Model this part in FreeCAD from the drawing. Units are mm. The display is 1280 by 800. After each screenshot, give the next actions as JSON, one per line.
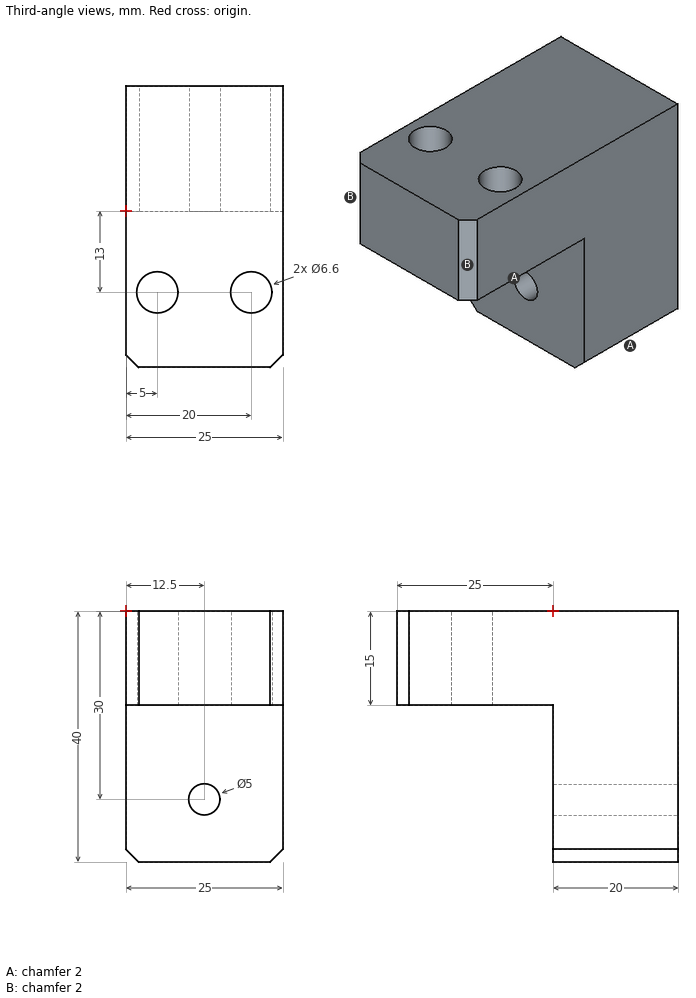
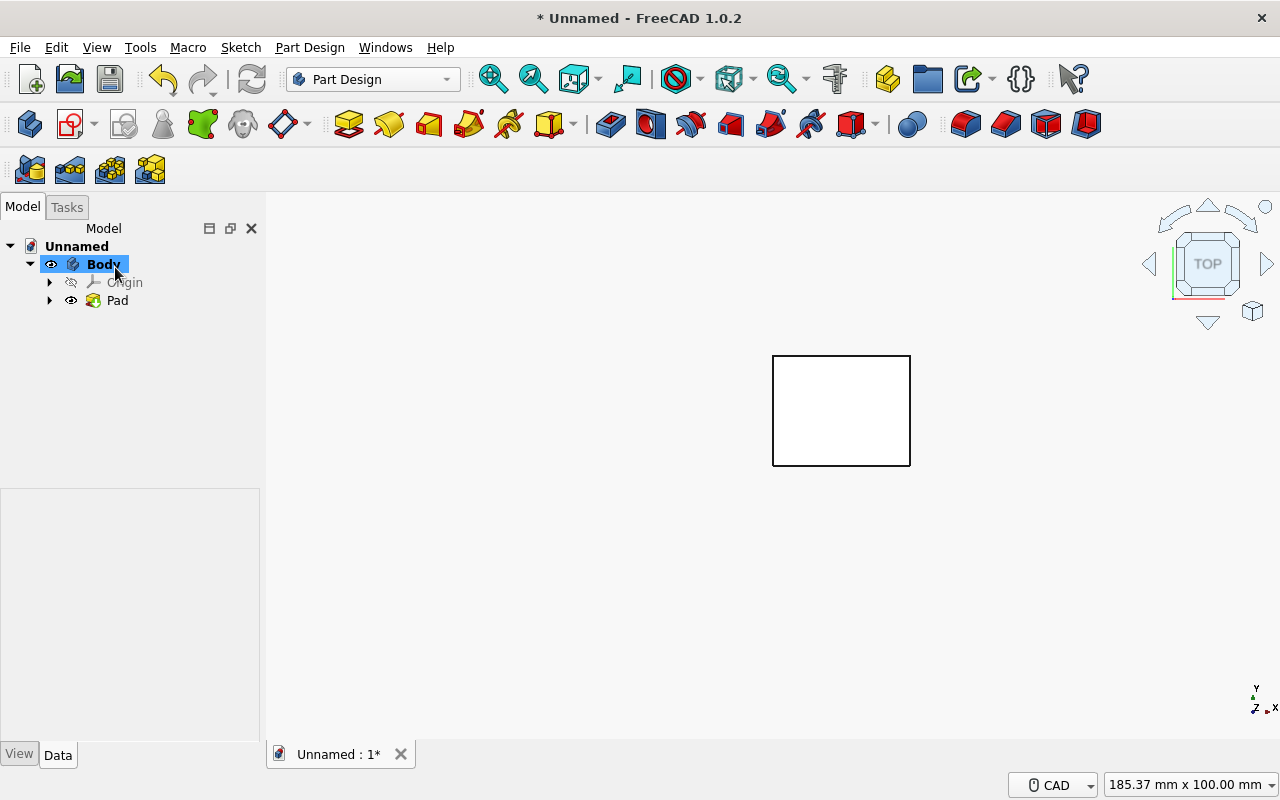
{"action": "key", "text": "v f"}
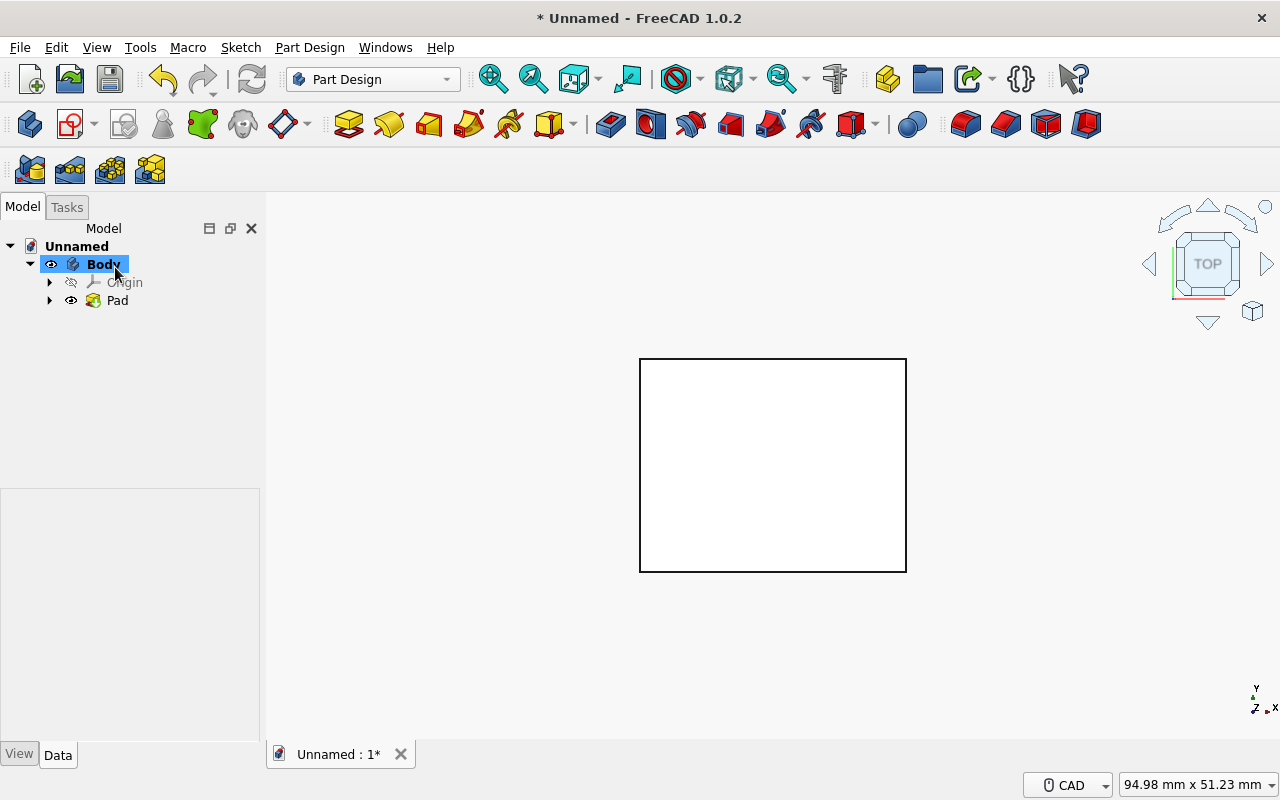
{"action": "key", "text": "1"}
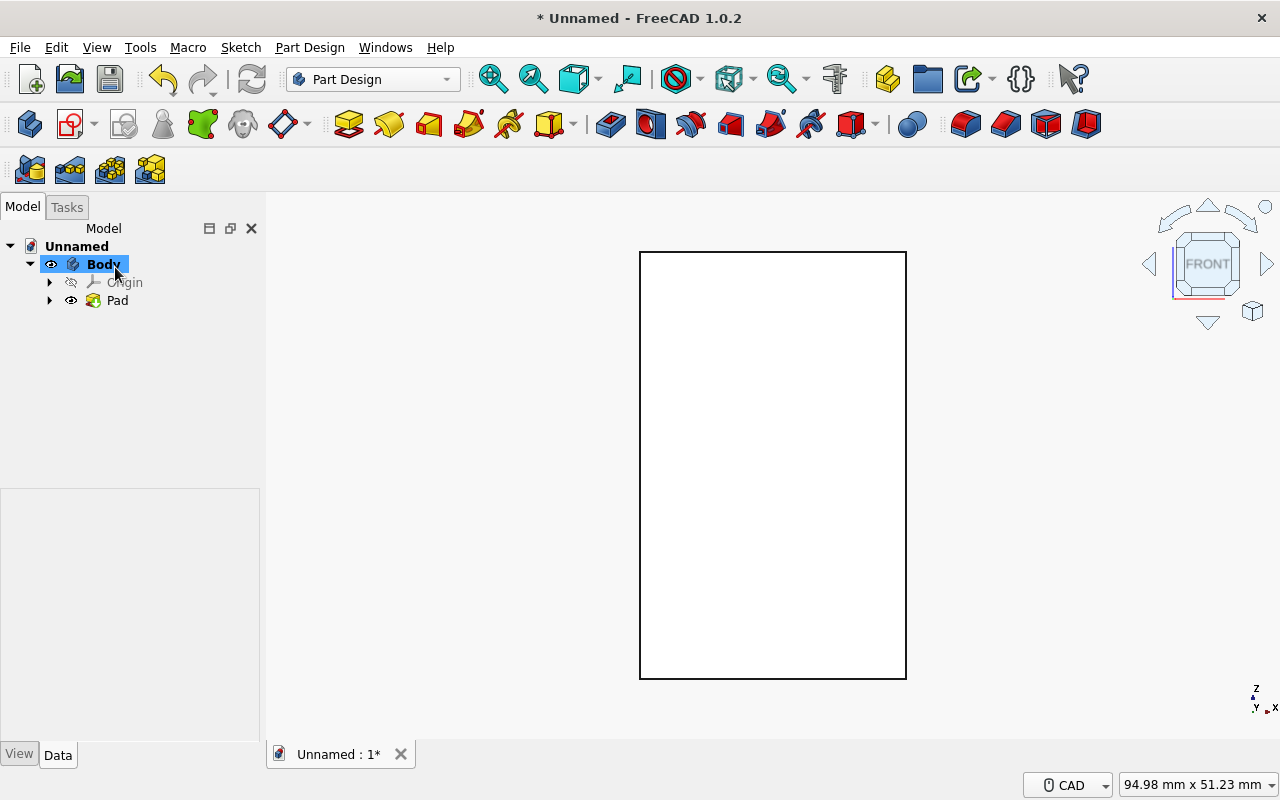
{"action": "key", "text": "3"}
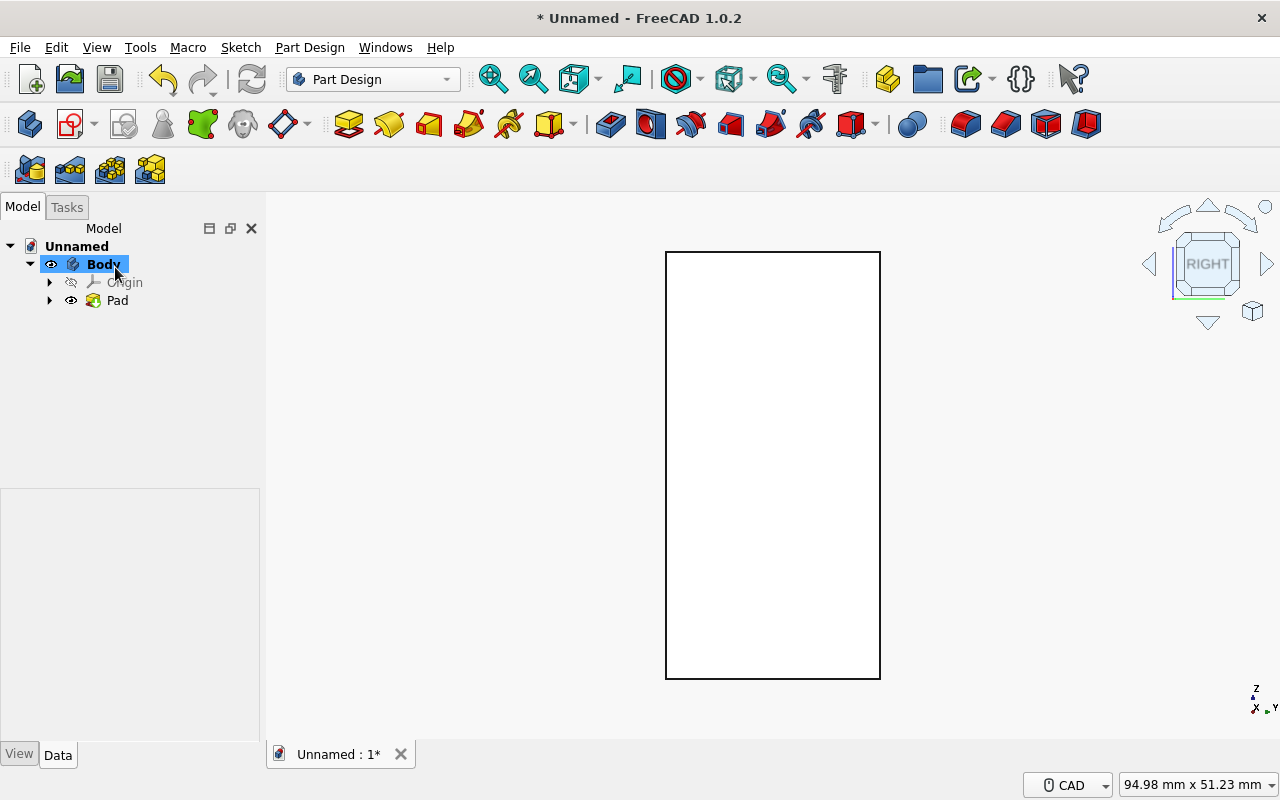
{"action": "left_click", "coordinate": [773, 678]}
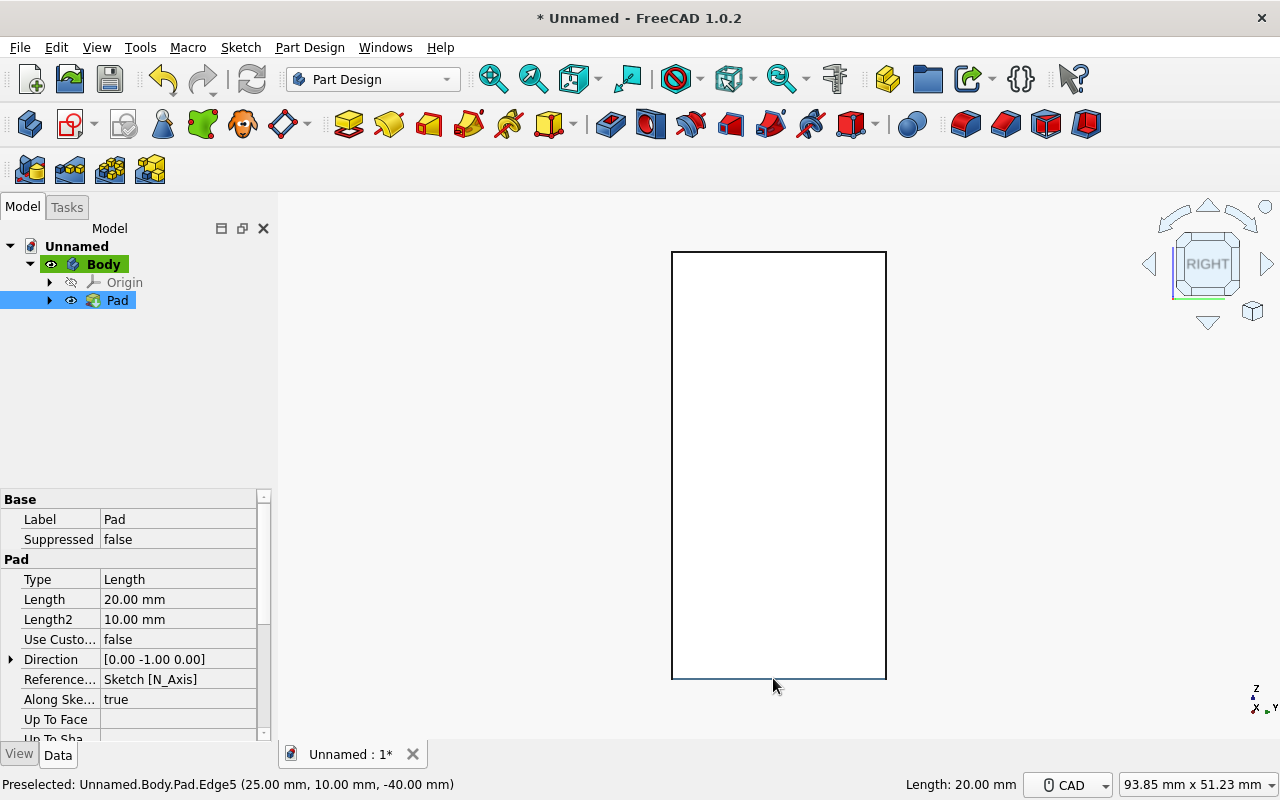
{"action": "key", "text": "5"}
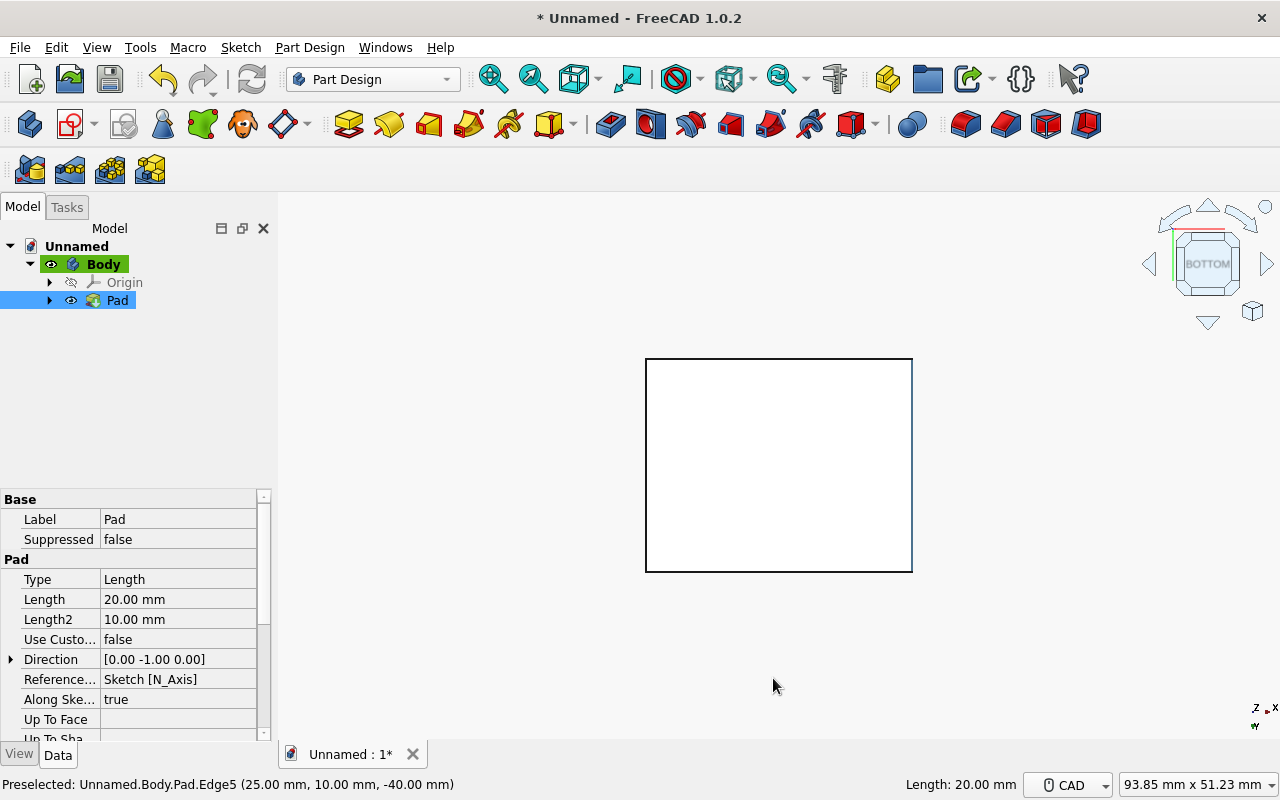
{"action": "key", "text": "v f"}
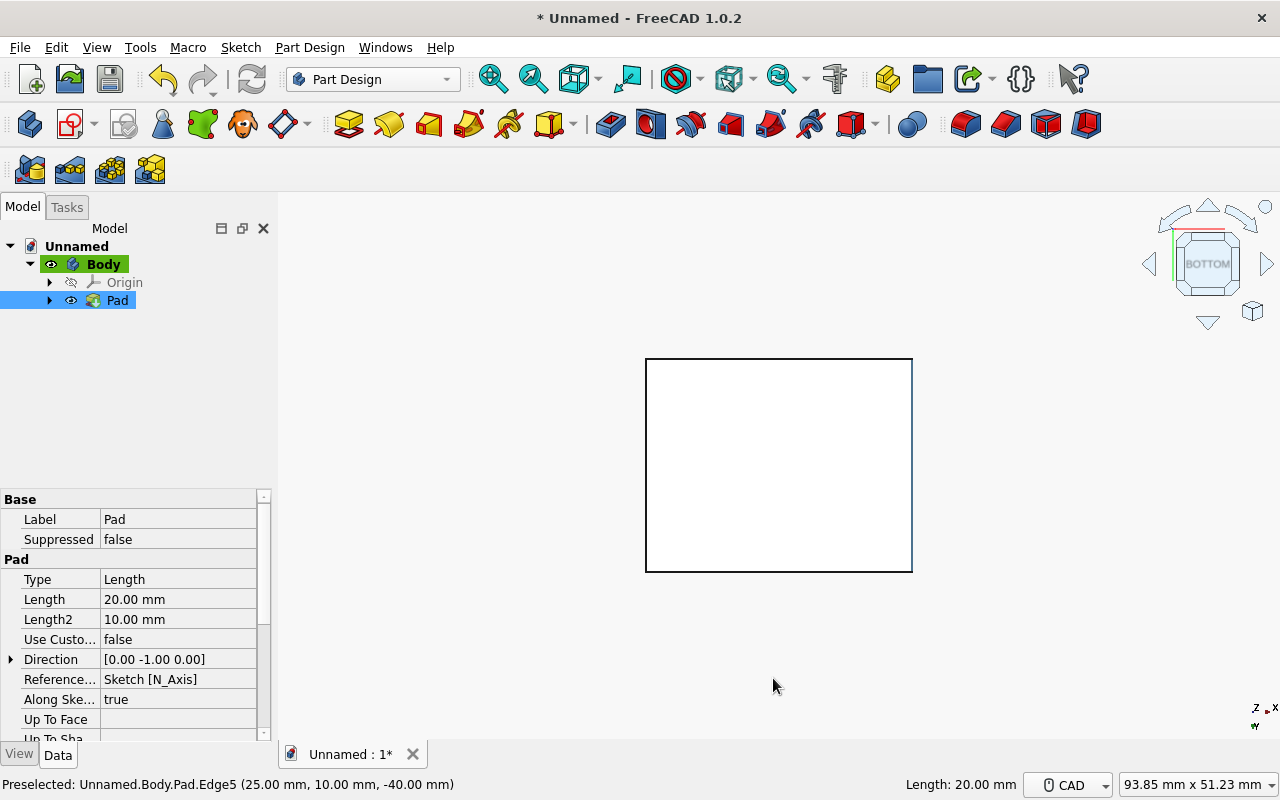
{"action": "left_click", "coordinate": [646, 464], "text": "ctrl"}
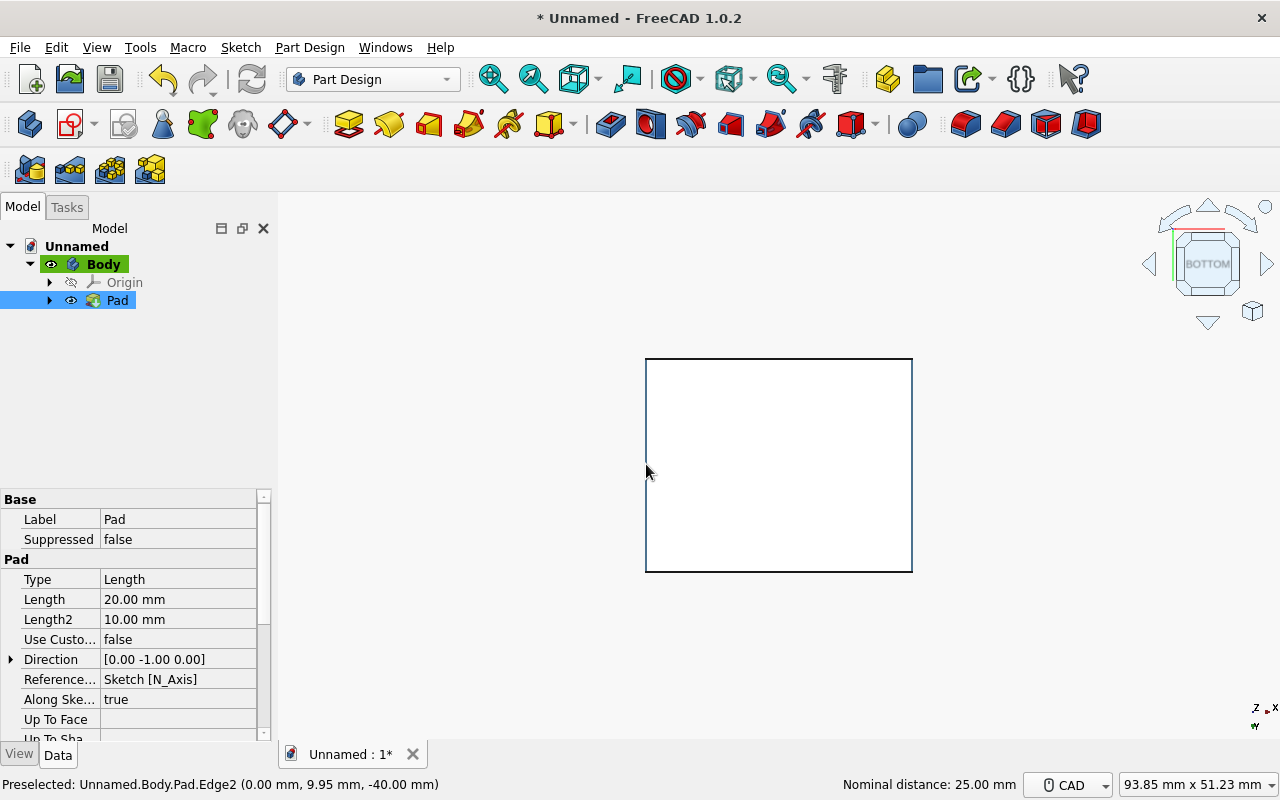
{"action": "left_click", "coordinate": [1006, 124]}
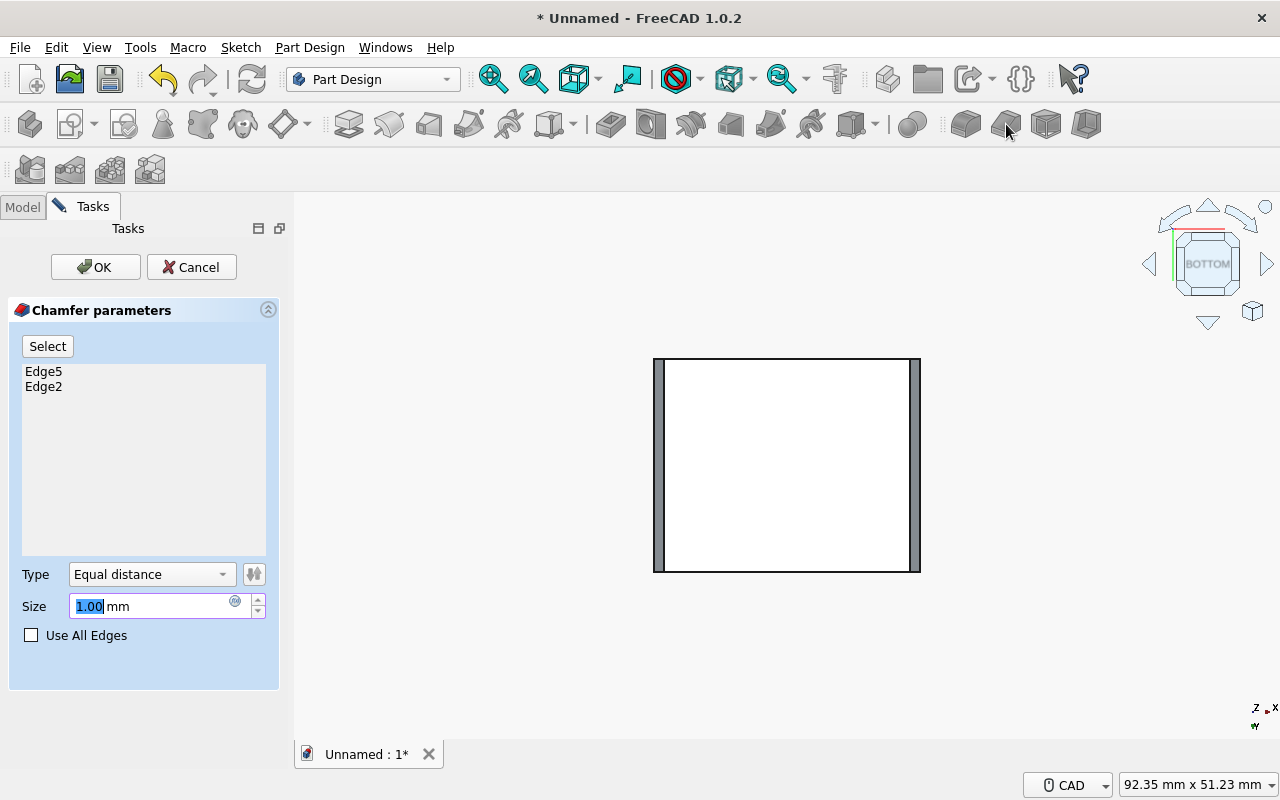
{"action": "type", "text": "2"}
{"action": "key", "text": "Tab"}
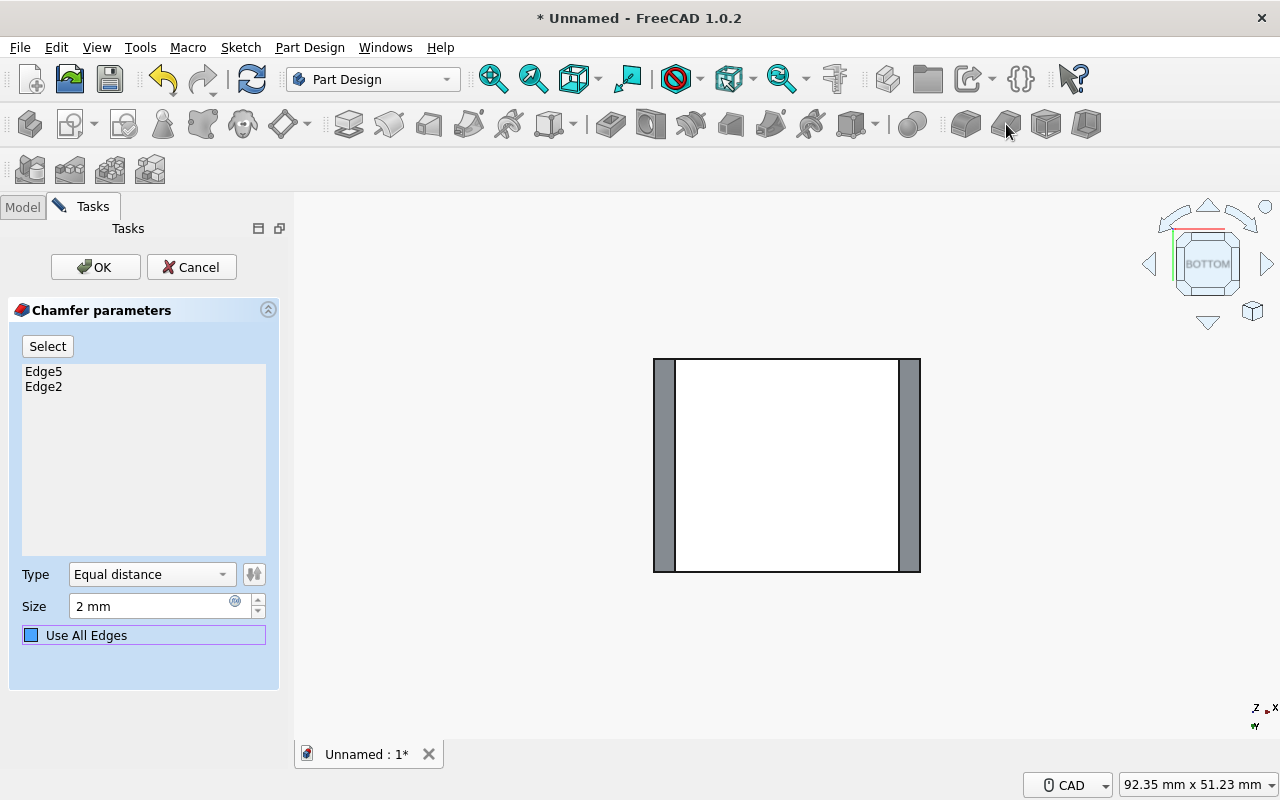
{"action": "left_click", "coordinate": [96, 267]}